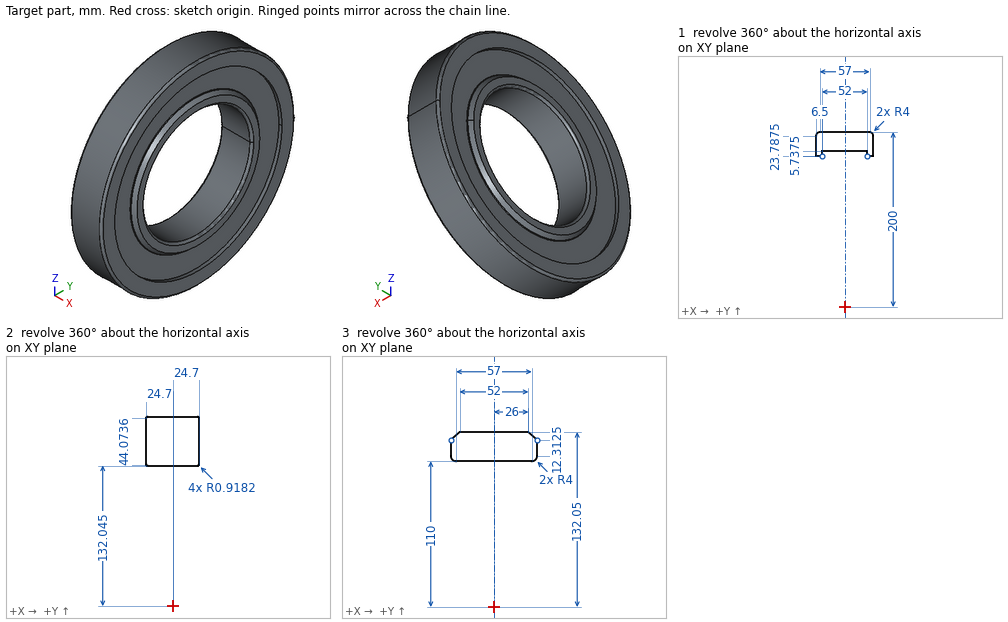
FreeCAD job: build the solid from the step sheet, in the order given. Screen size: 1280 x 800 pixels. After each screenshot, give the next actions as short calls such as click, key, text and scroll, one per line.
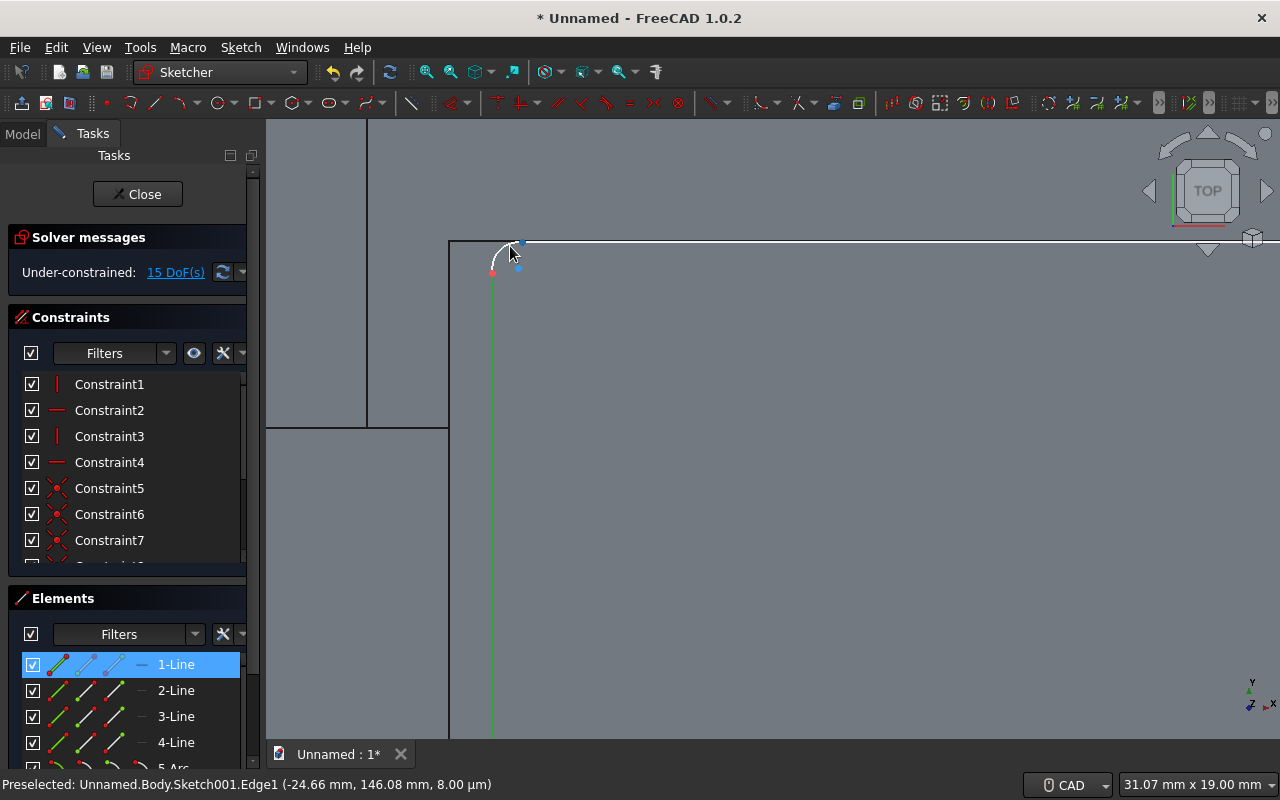
click(508, 245)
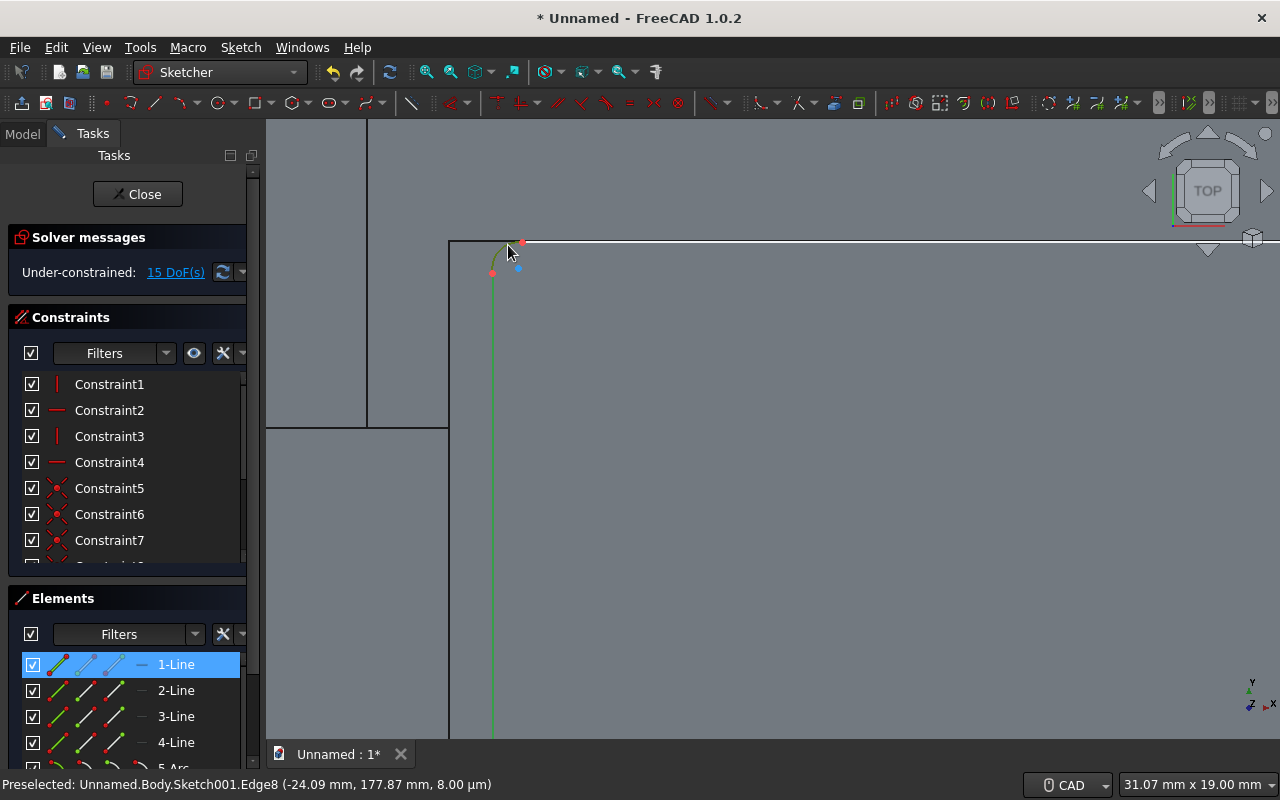
click(606, 104)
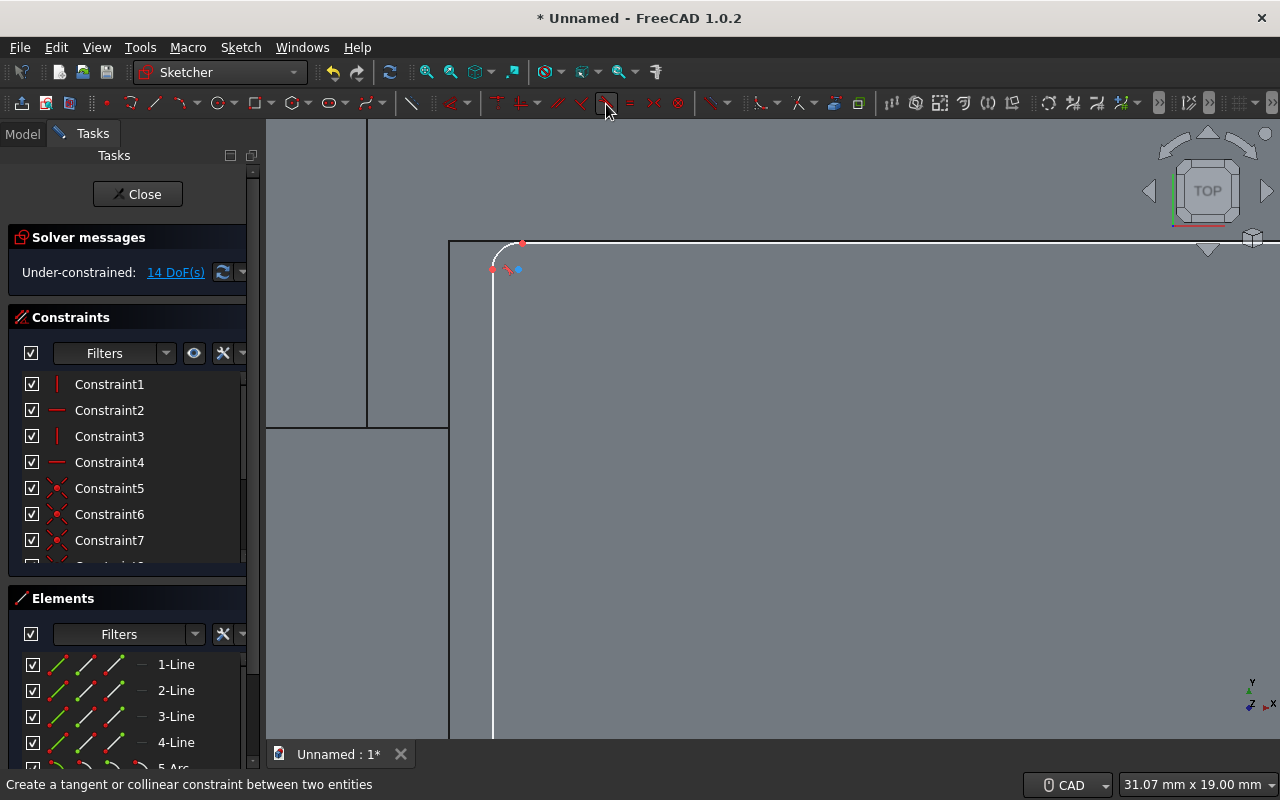
scroll(510, 246, down, 7)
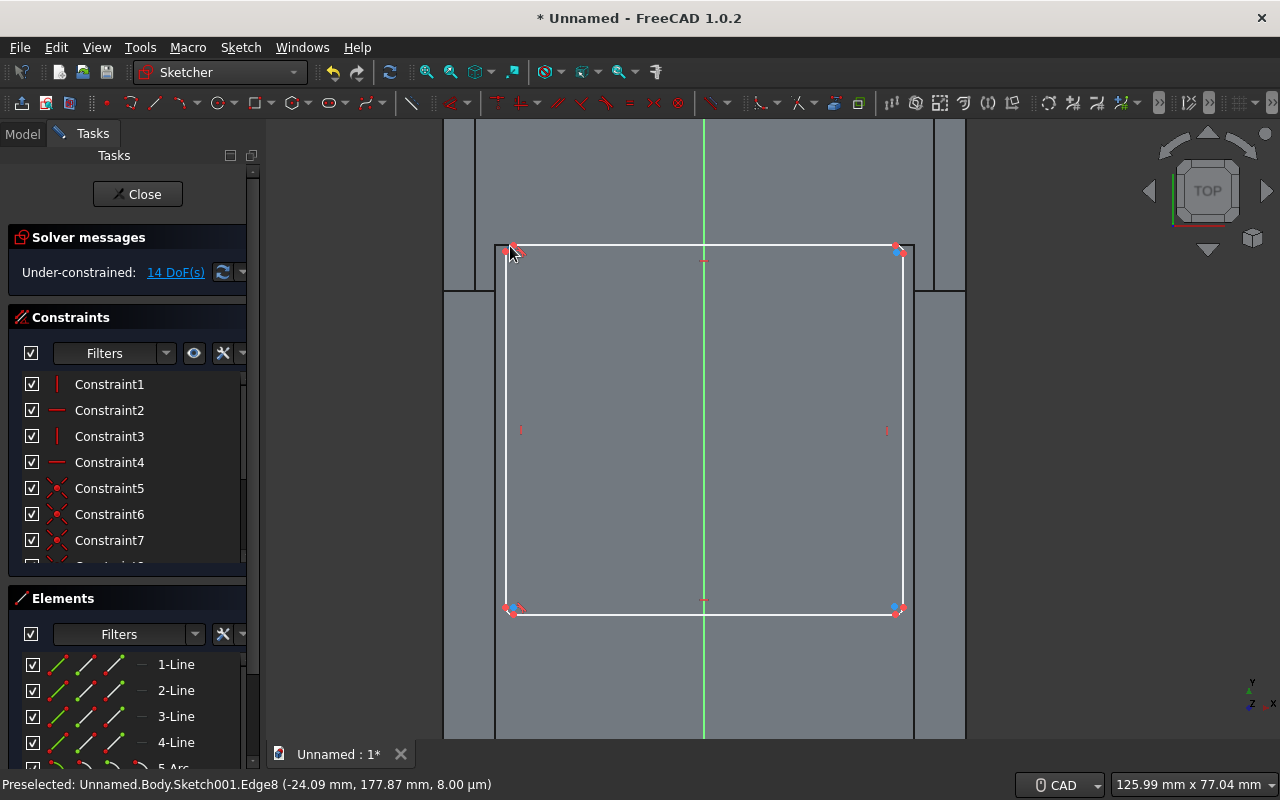
click(628, 615)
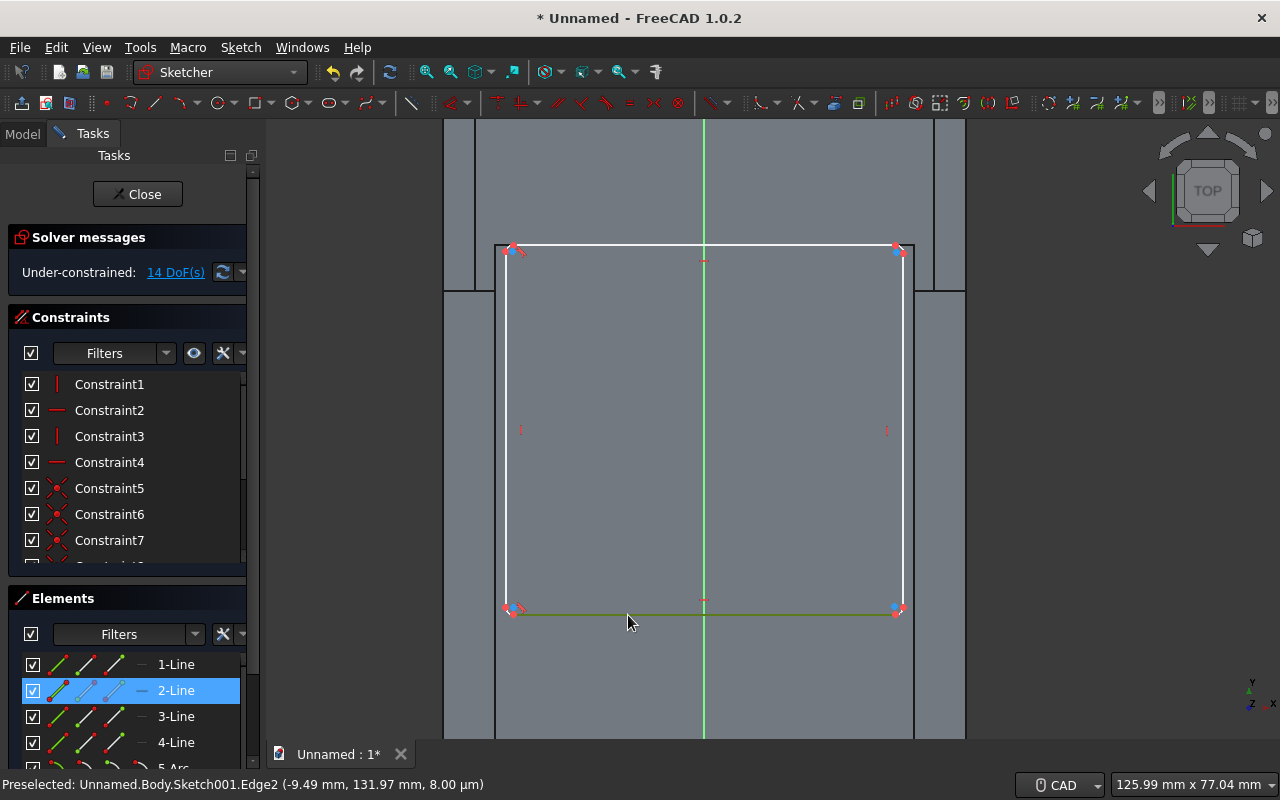
scroll(508, 612, up, 5)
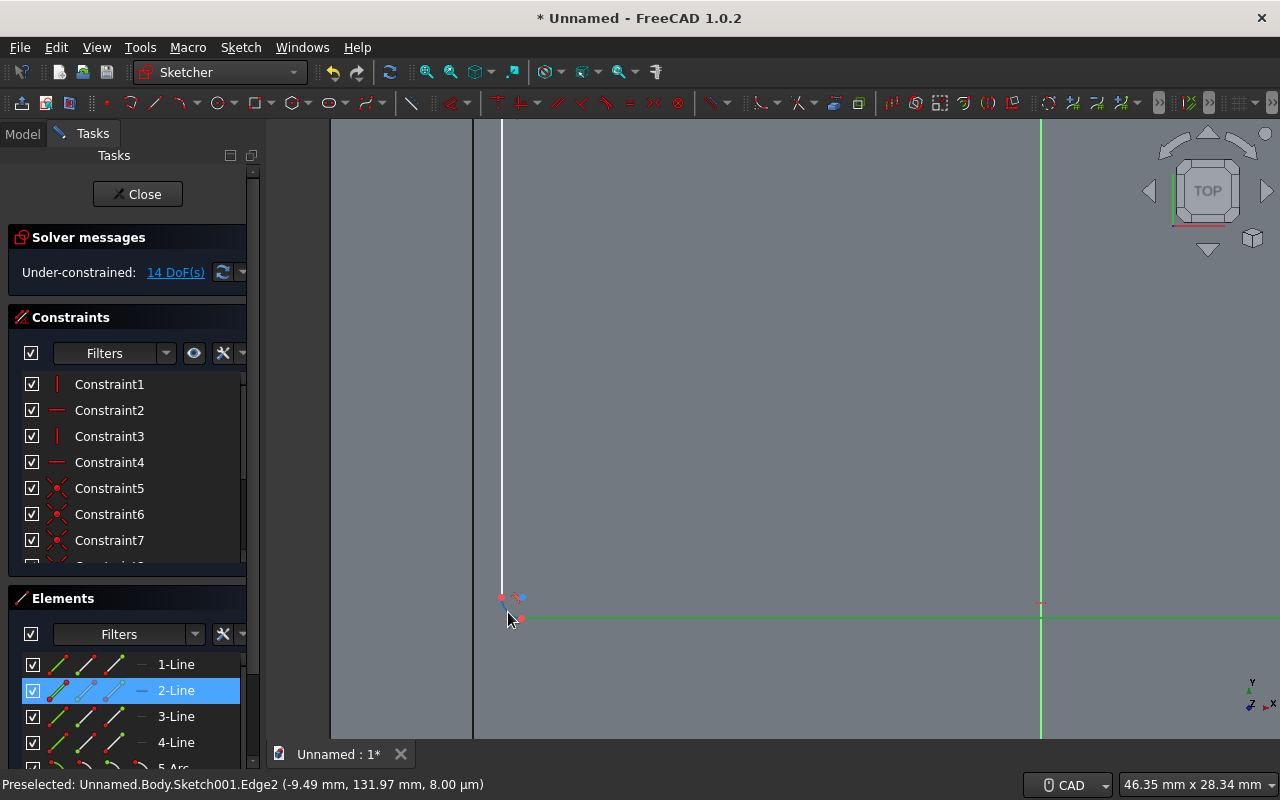
click(507, 612)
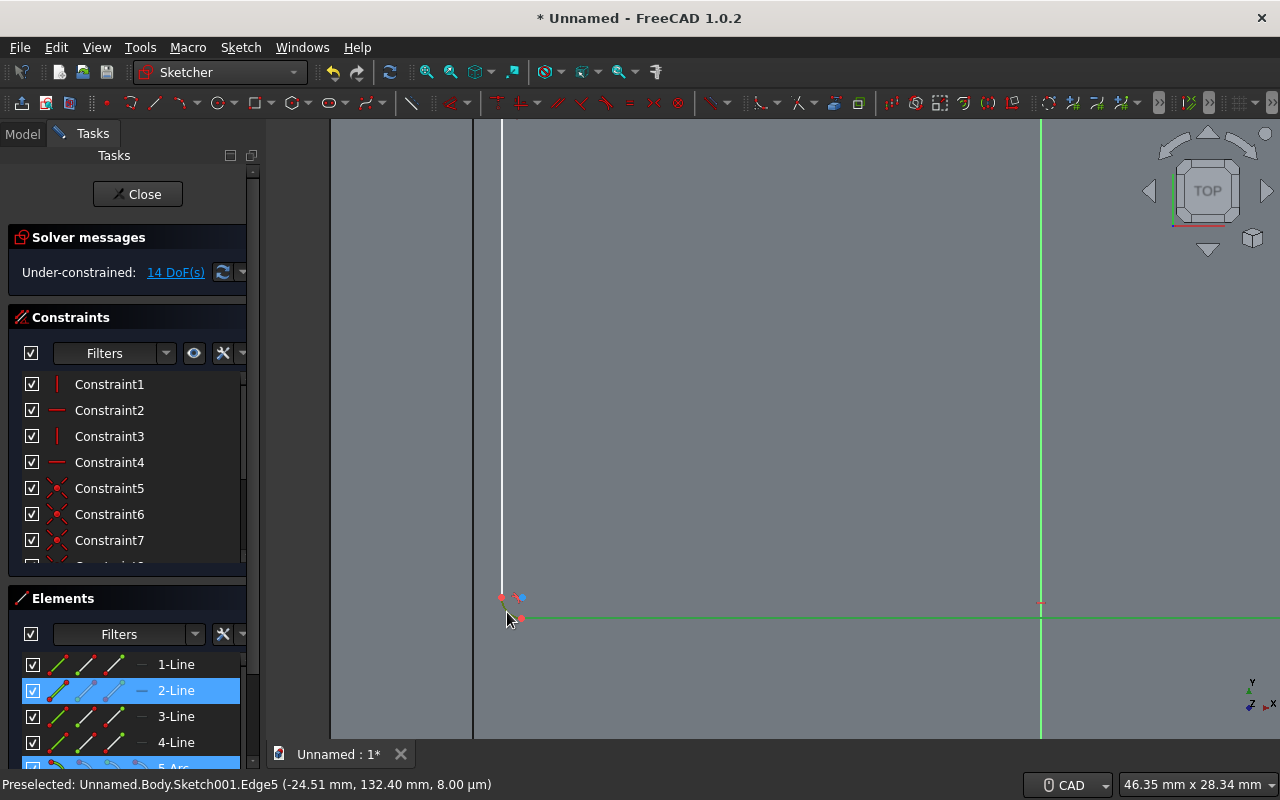
click(606, 104)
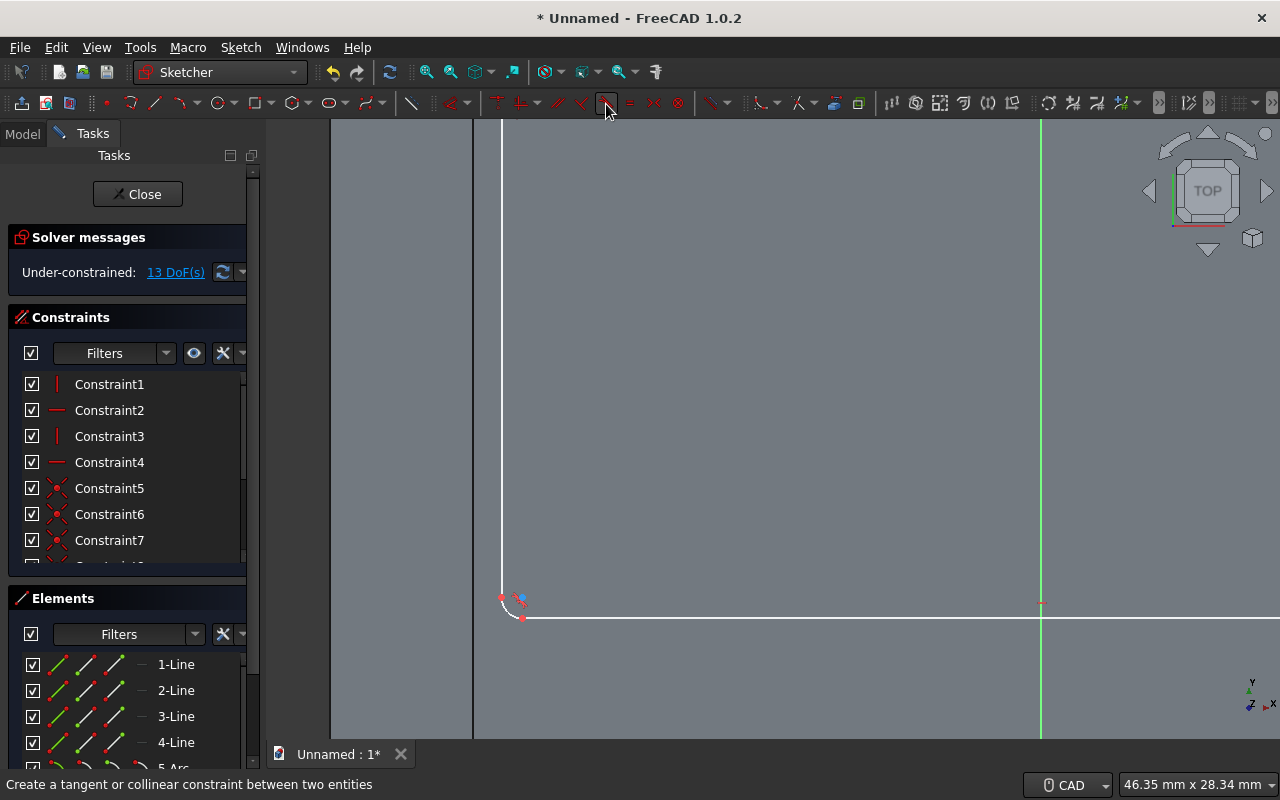
click(834, 618)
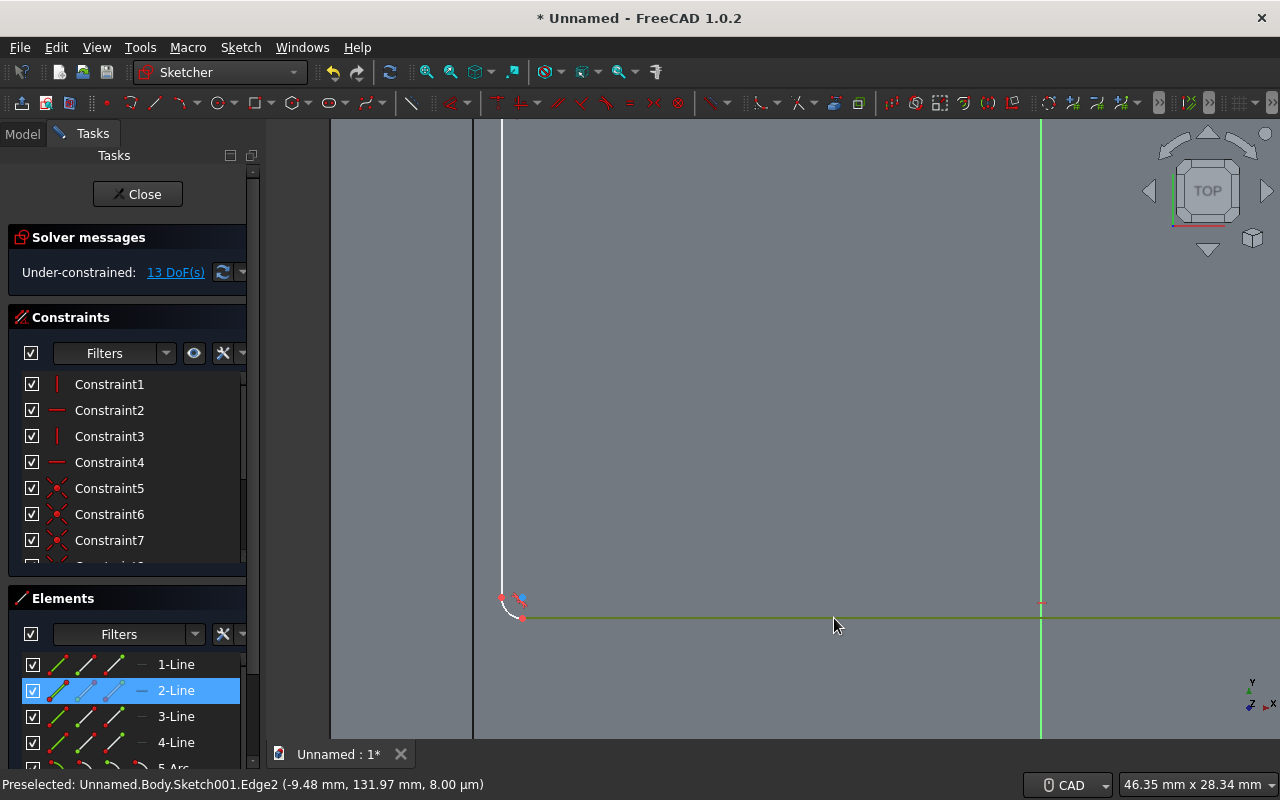
scroll(508, 612, down, 5)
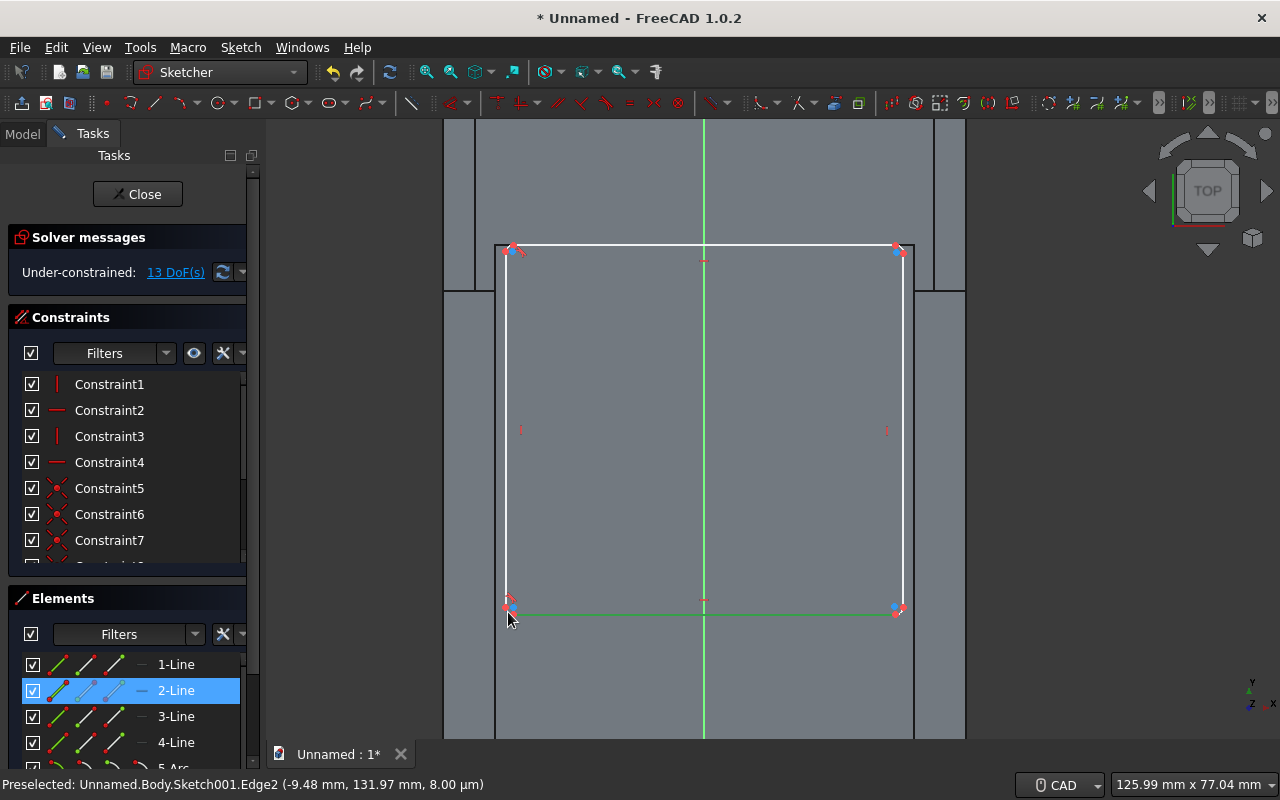
scroll(899, 614, up, 8)